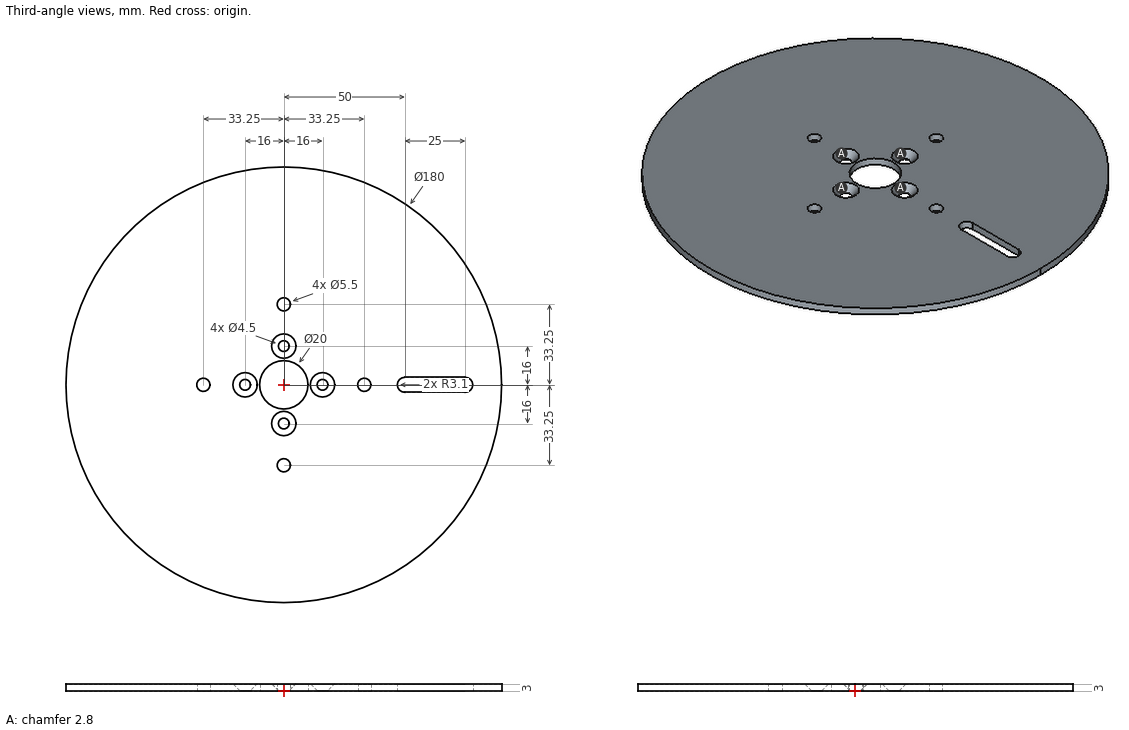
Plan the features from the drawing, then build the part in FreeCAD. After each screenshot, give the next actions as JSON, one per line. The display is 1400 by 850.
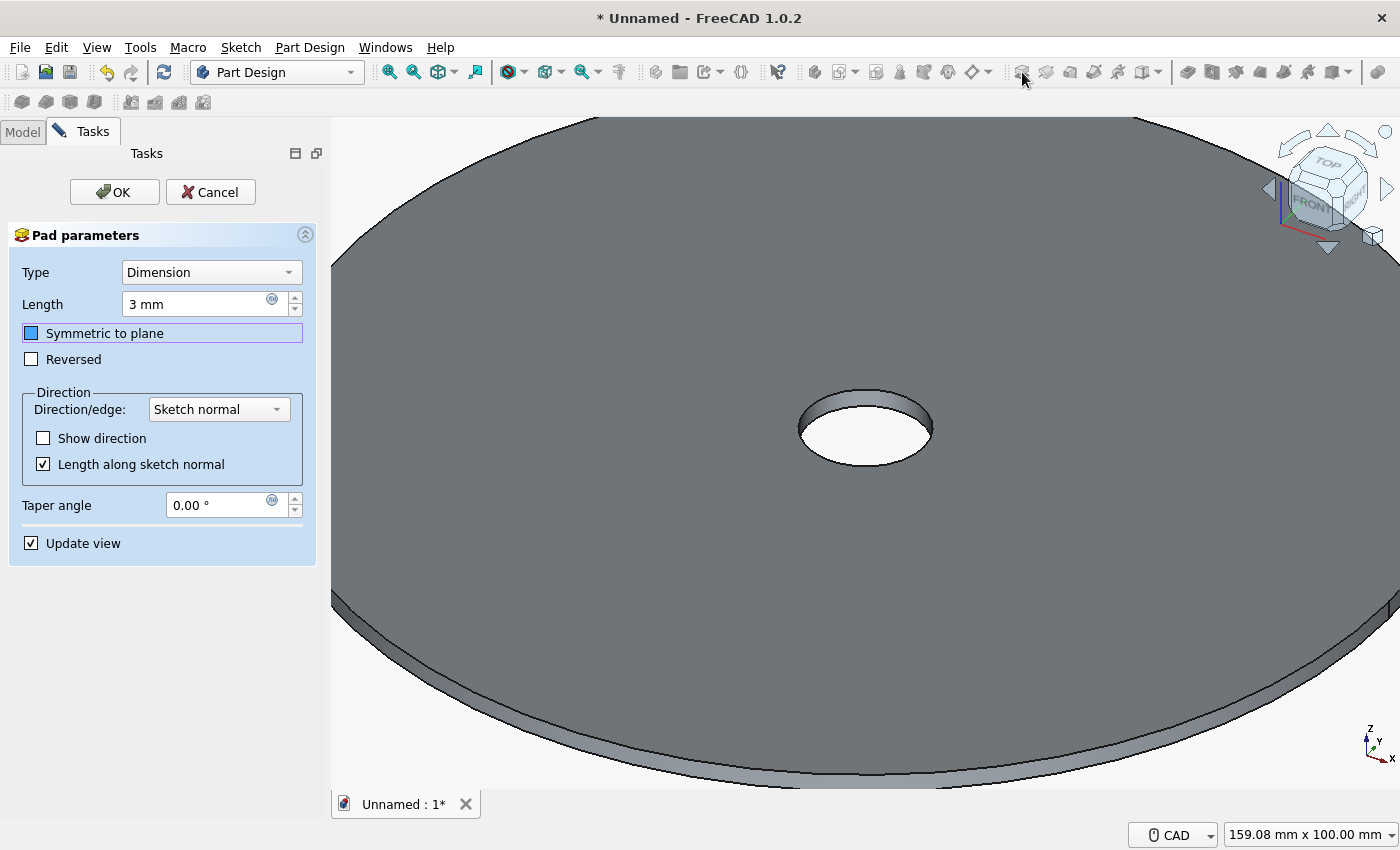
{"action": "left_click", "coordinate": [115, 192]}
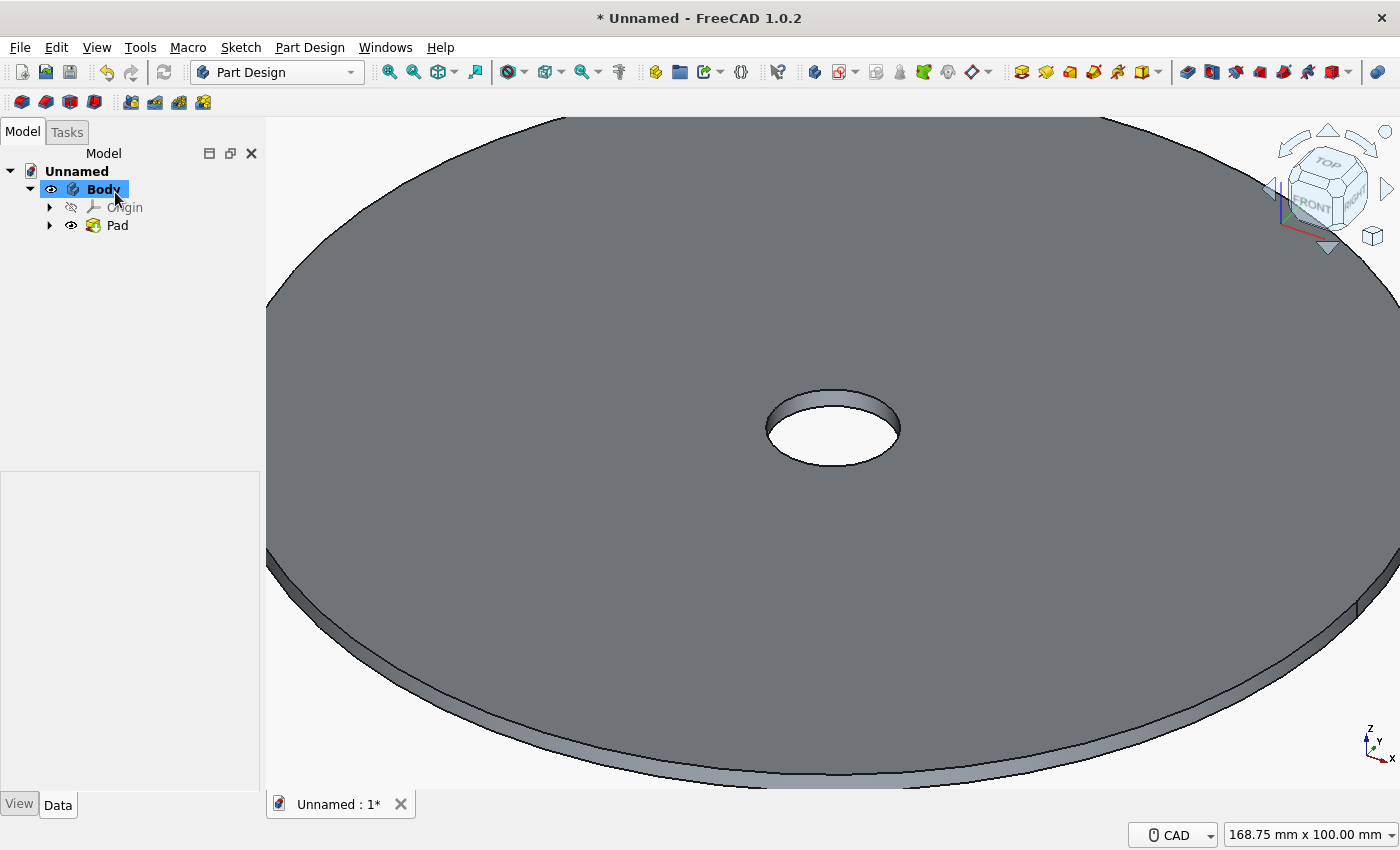
{"action": "left_click", "coordinate": [390, 72]}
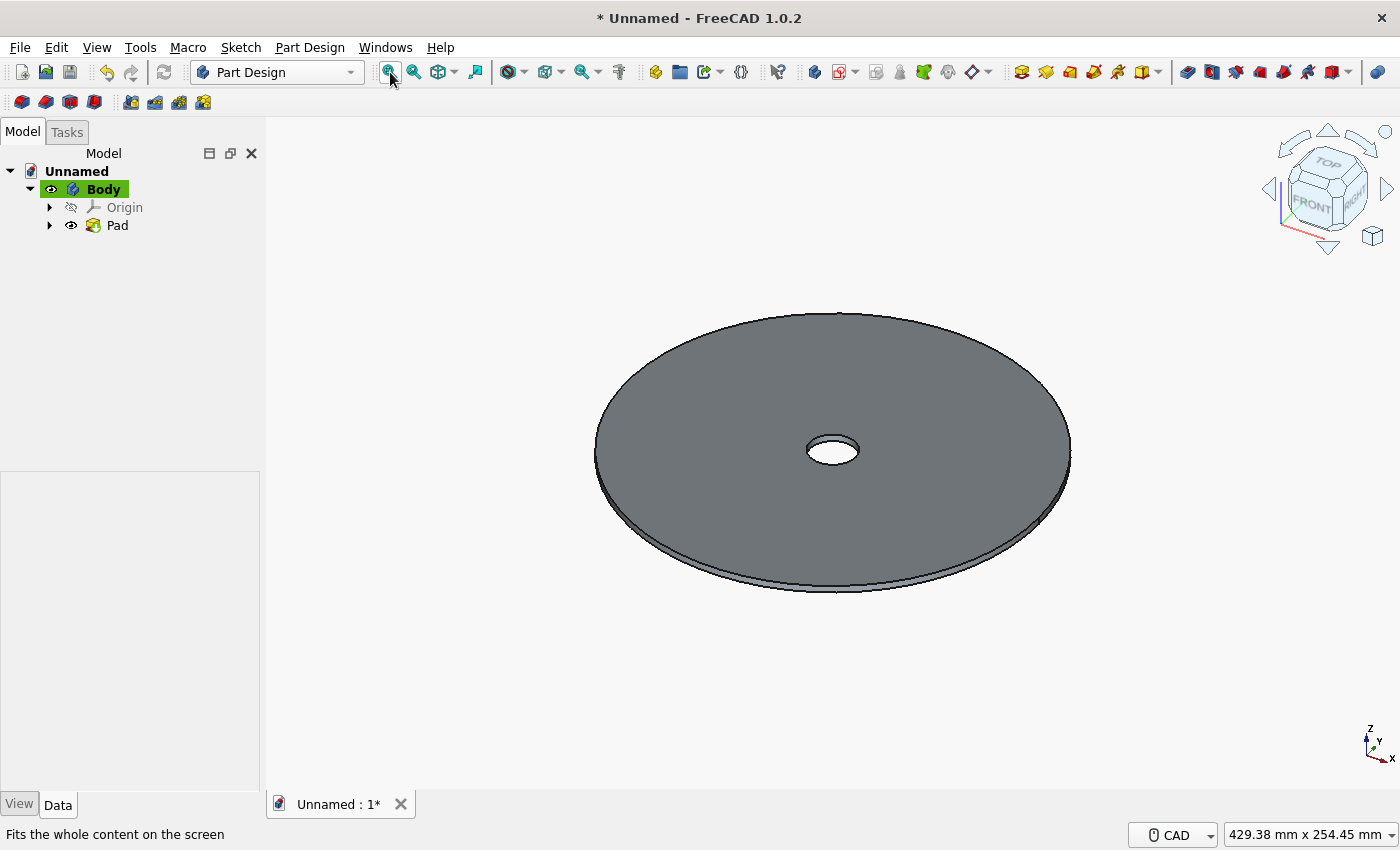
{"action": "left_click", "coordinate": [950, 488]}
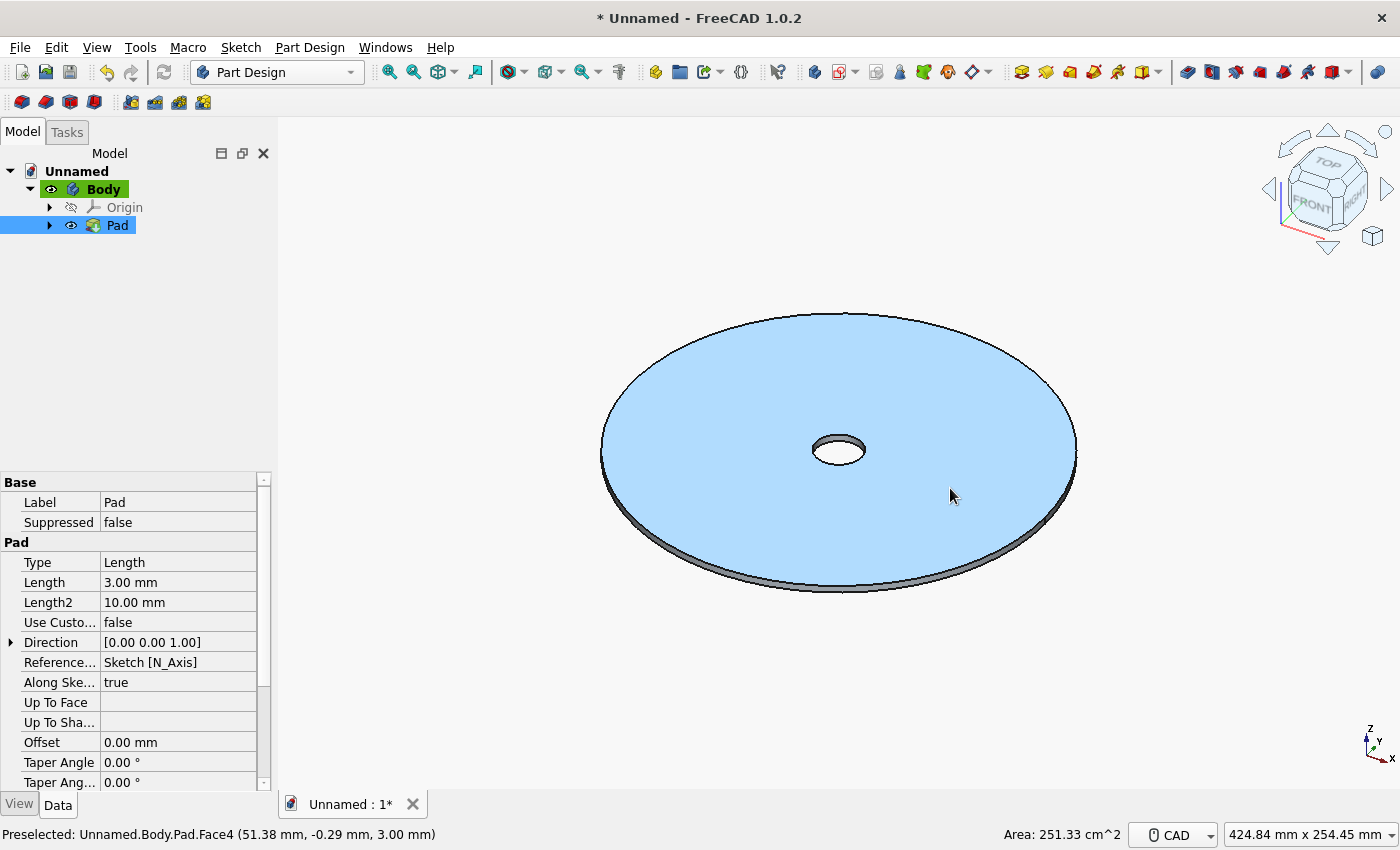
{"action": "left_click", "coordinate": [840, 72]}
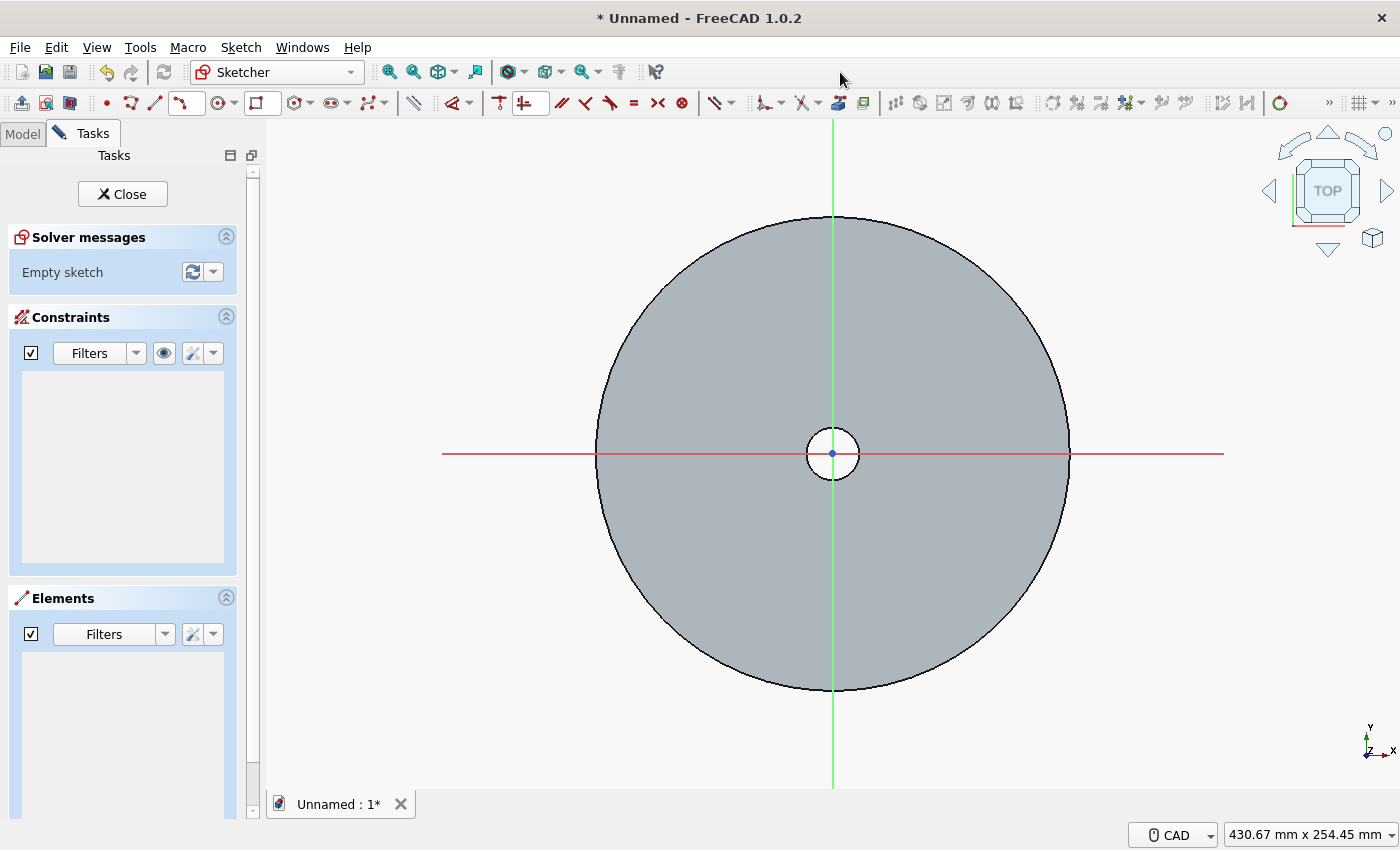
{"action": "scroll", "coordinate": [989, 454], "scroll_direction": "up", "scroll_amount": 4}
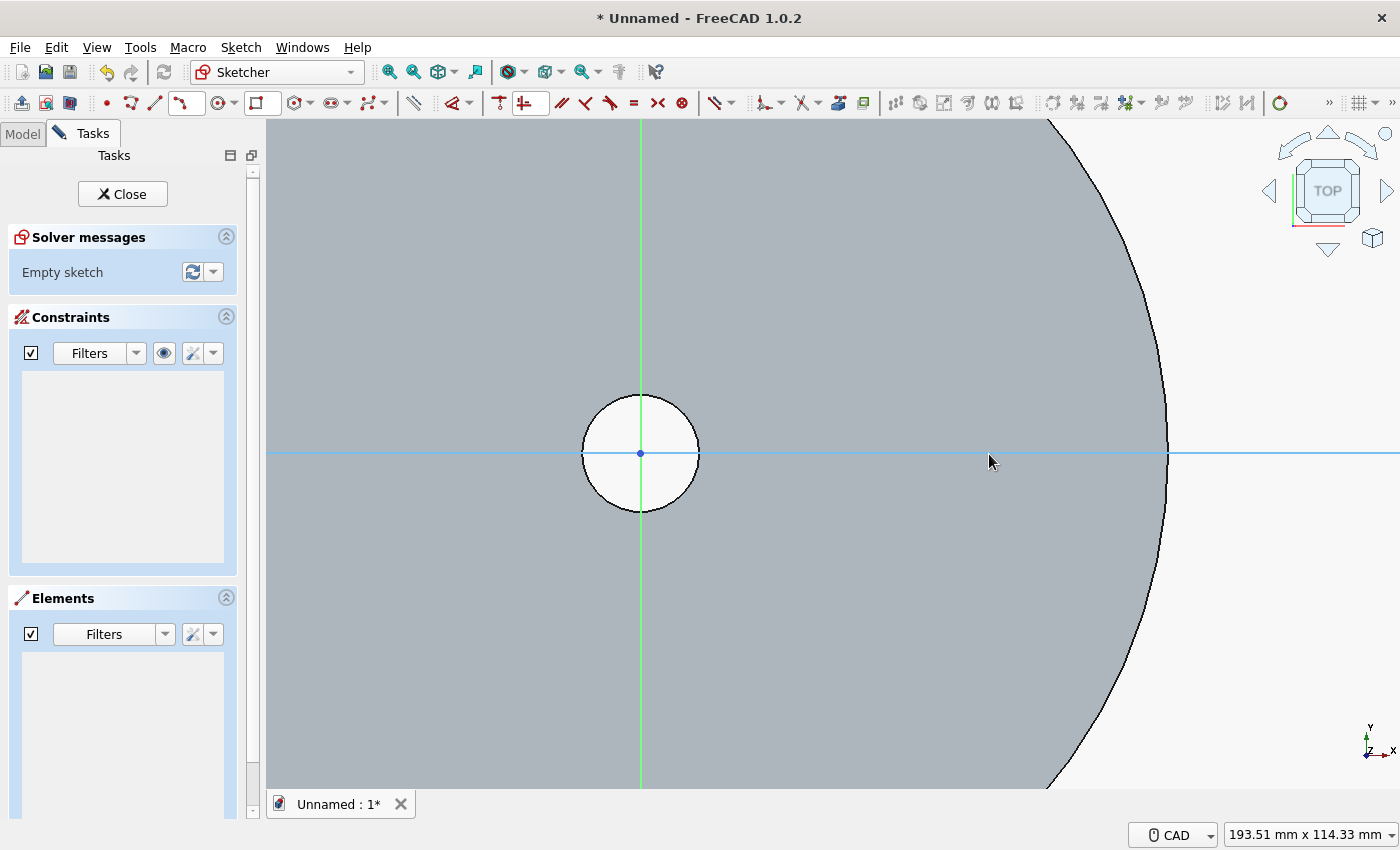
{"action": "left_click", "coordinate": [332, 104]}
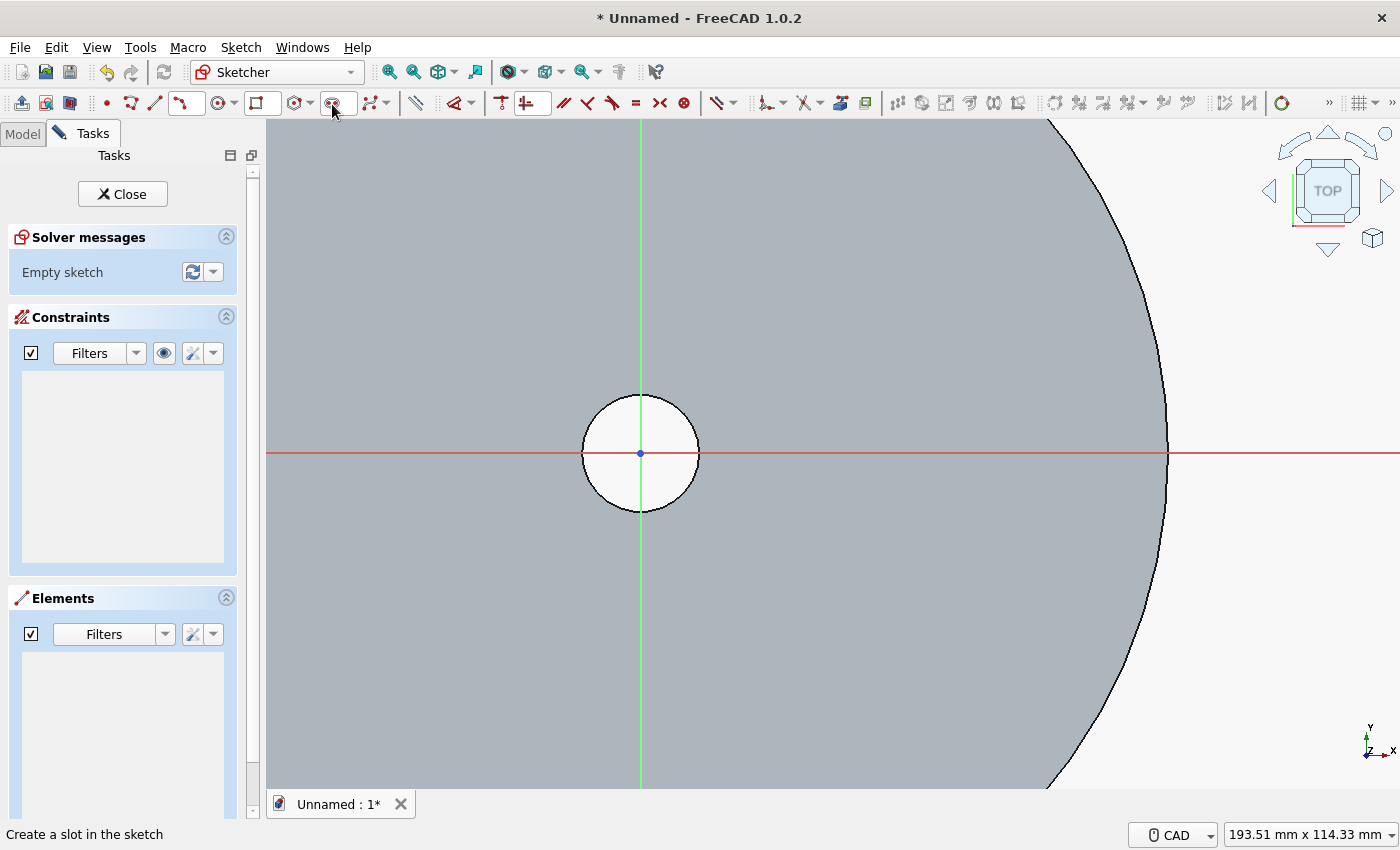
{"action": "scroll", "coordinate": [934, 453], "scroll_direction": "up", "scroll_amount": 2}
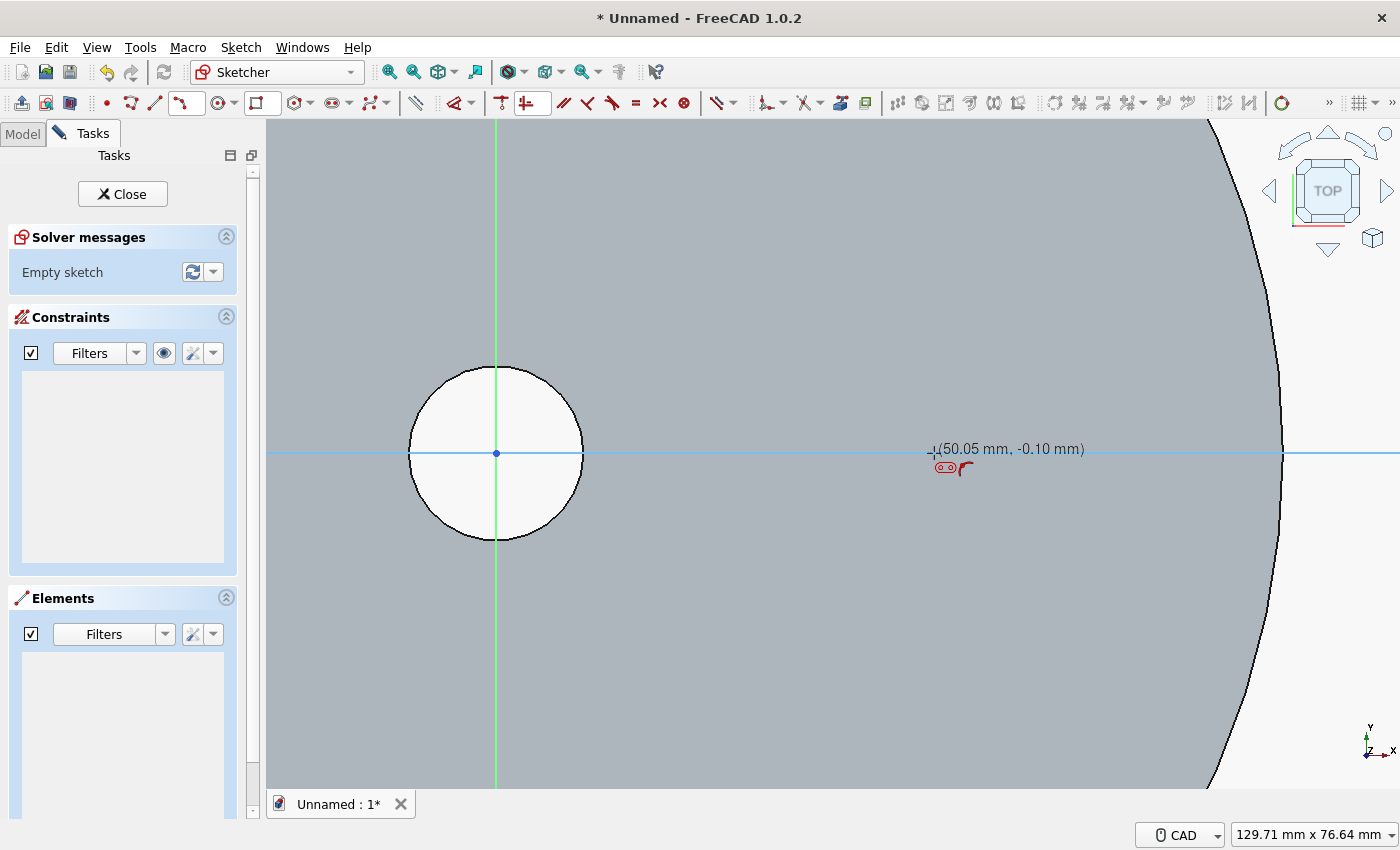
{"action": "left_click", "coordinate": [933, 453]}